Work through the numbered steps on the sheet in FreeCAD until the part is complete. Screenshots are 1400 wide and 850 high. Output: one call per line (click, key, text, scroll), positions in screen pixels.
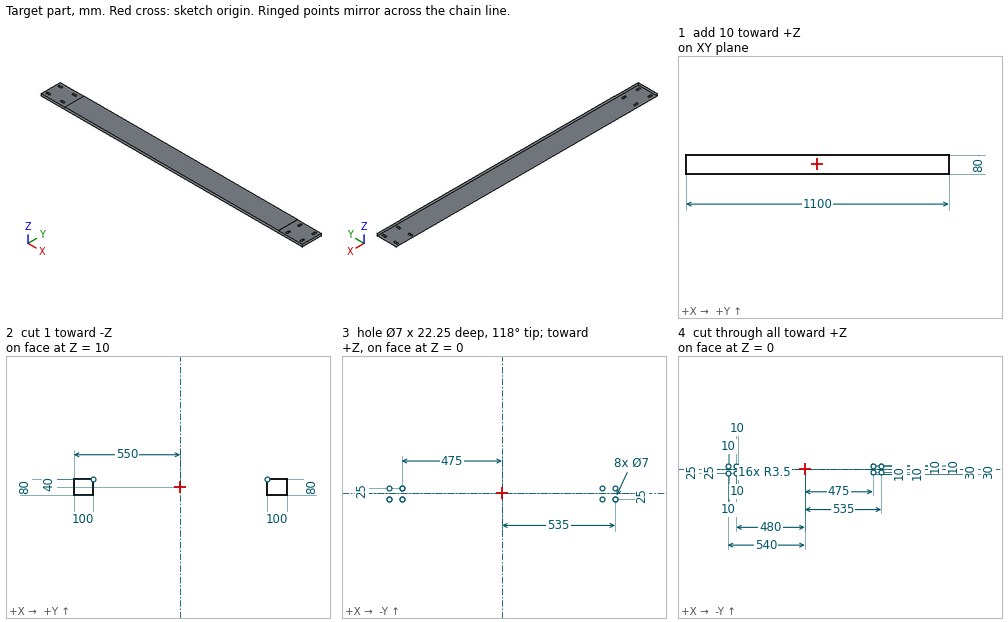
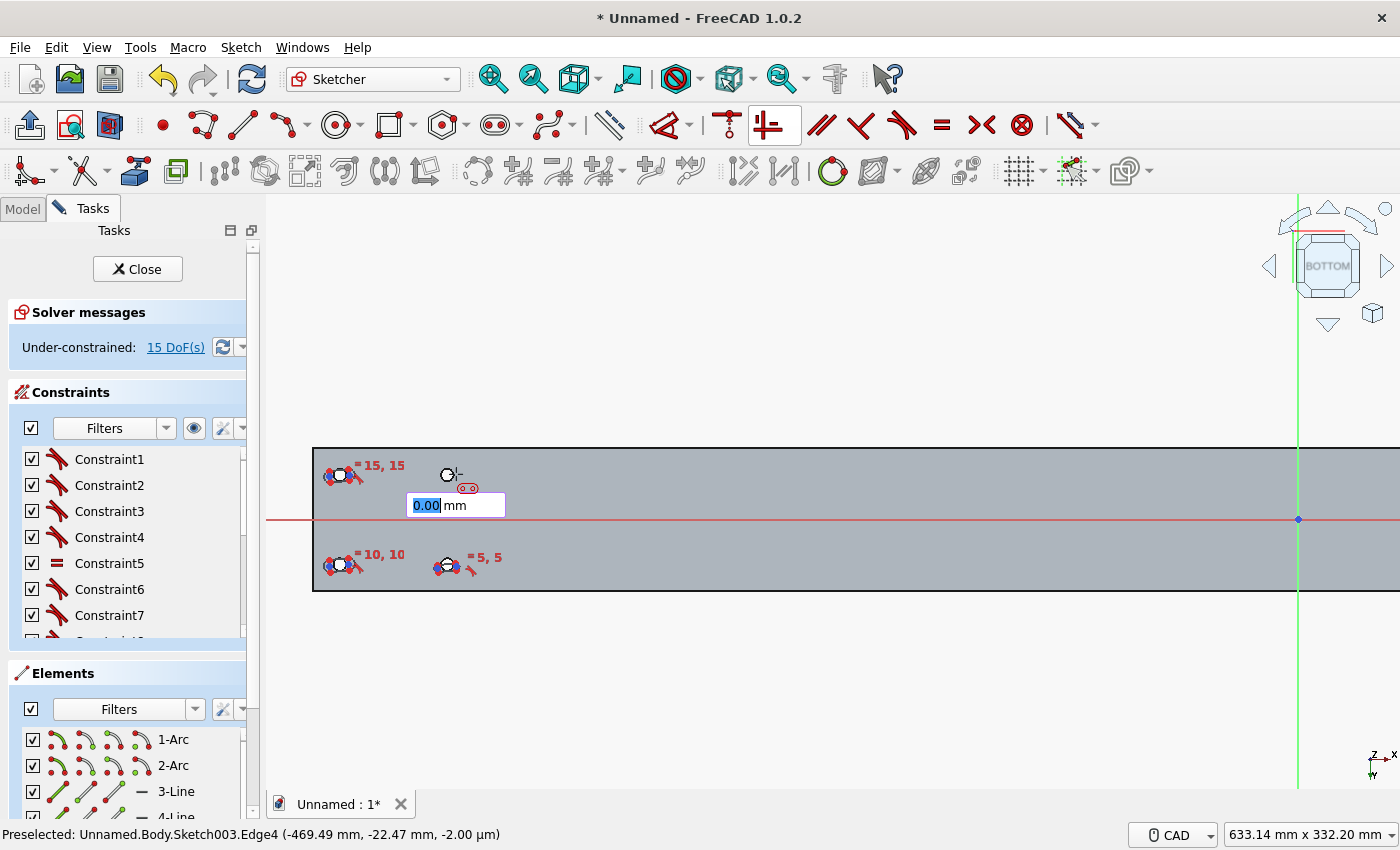
scroll(447, 481, up, 5)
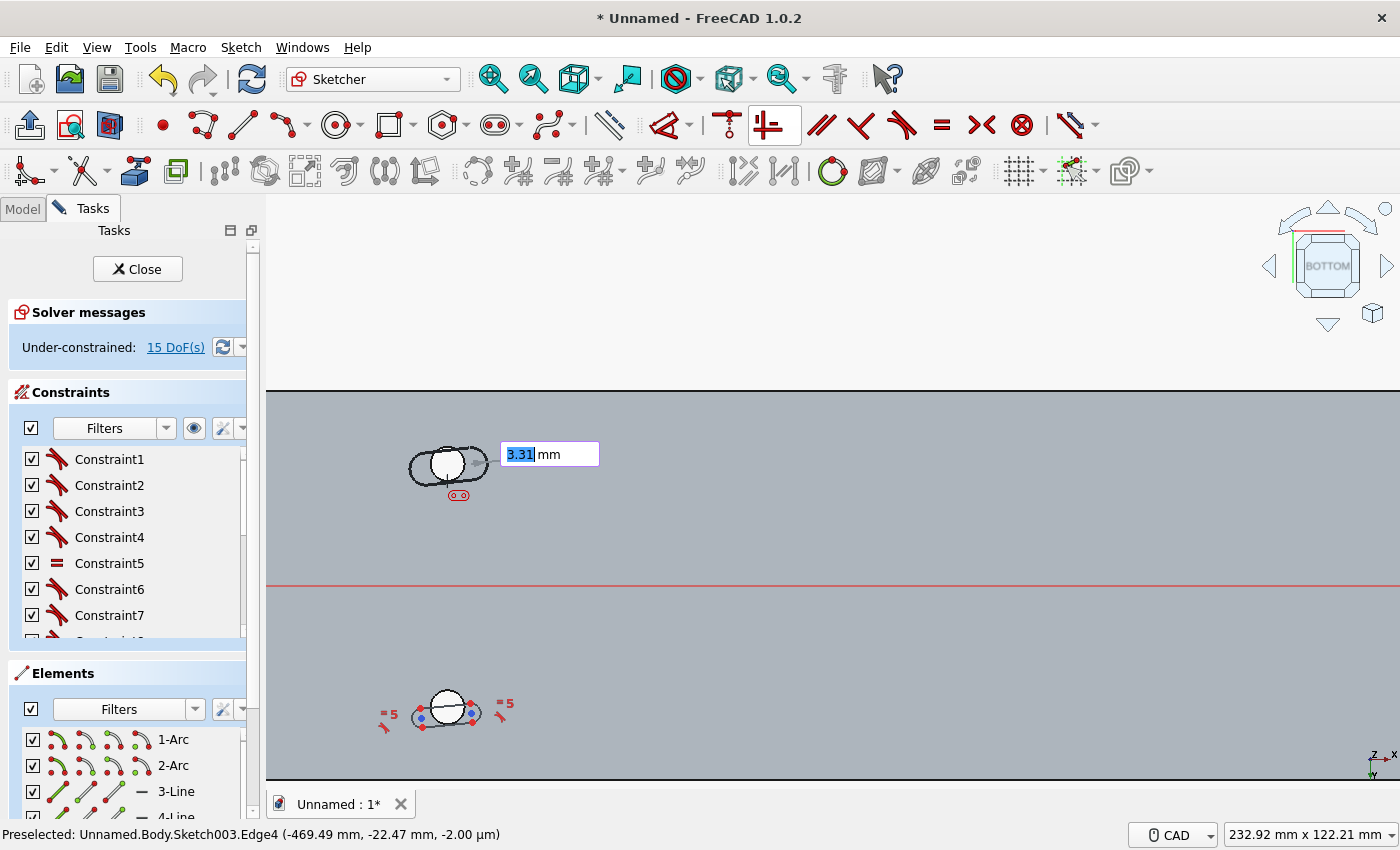
click(448, 481)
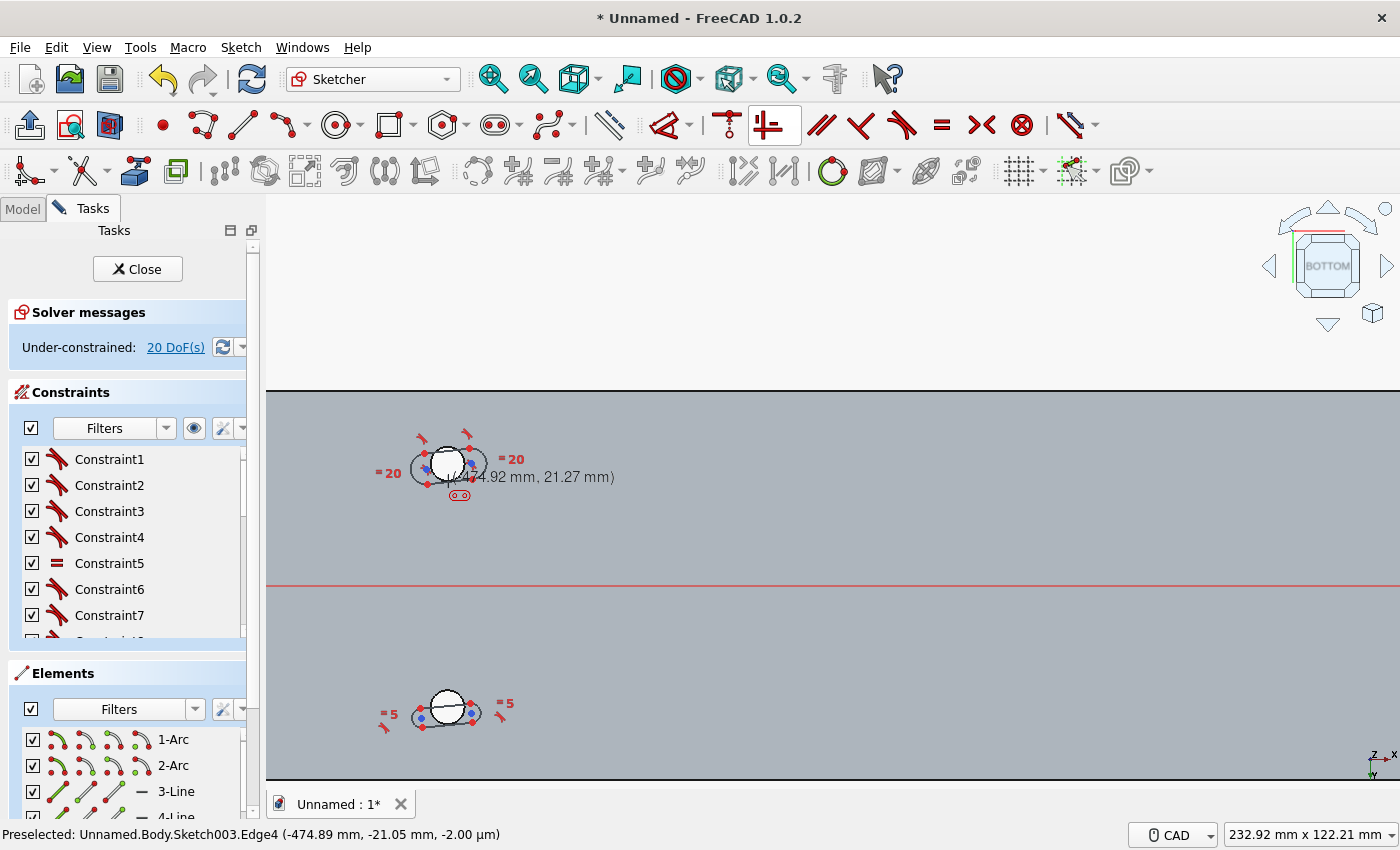
scroll(454, 477, down, 10)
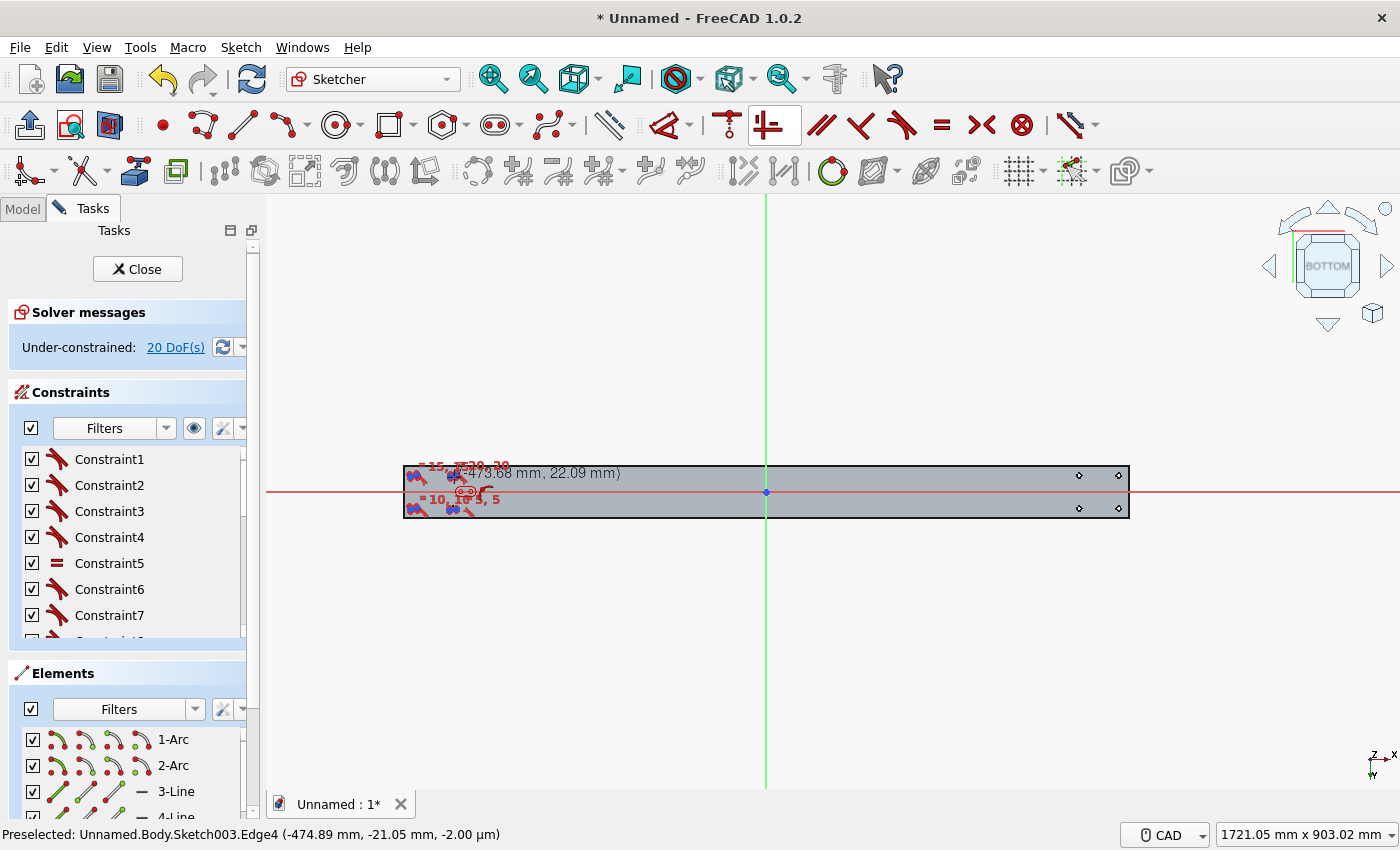
scroll(1119, 512, up, 12)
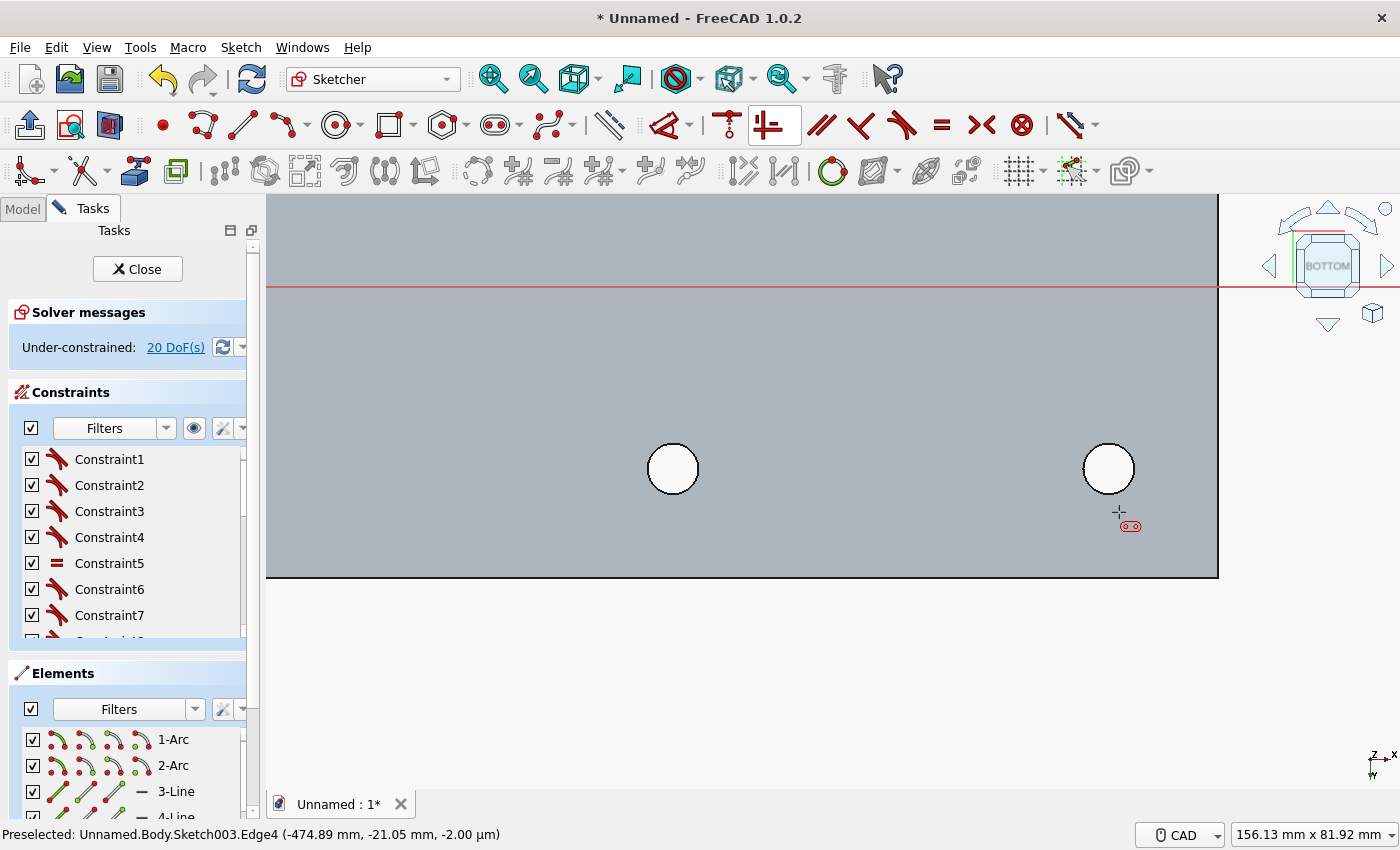
scroll(1120, 512, down, 12)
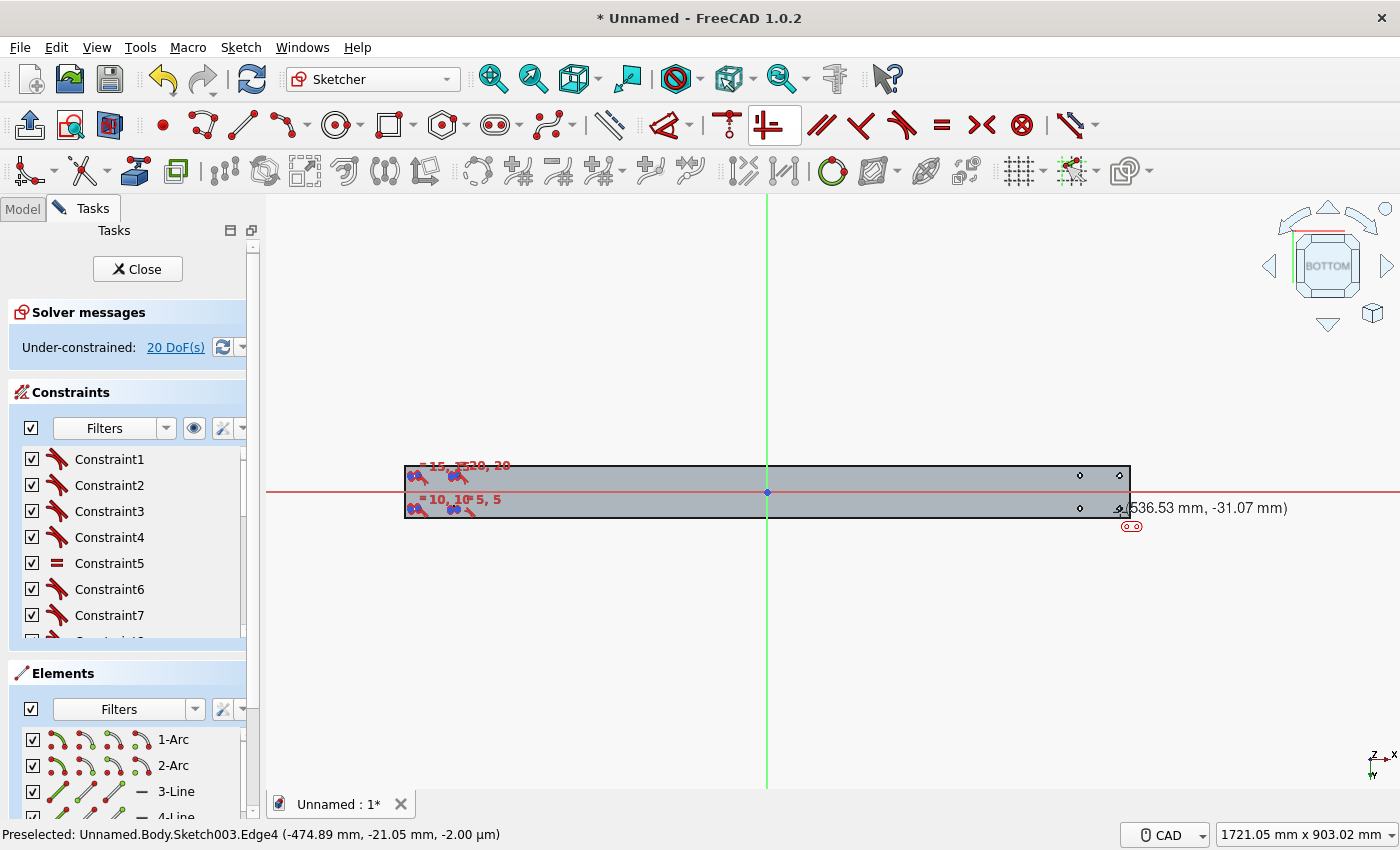
click(1120, 512)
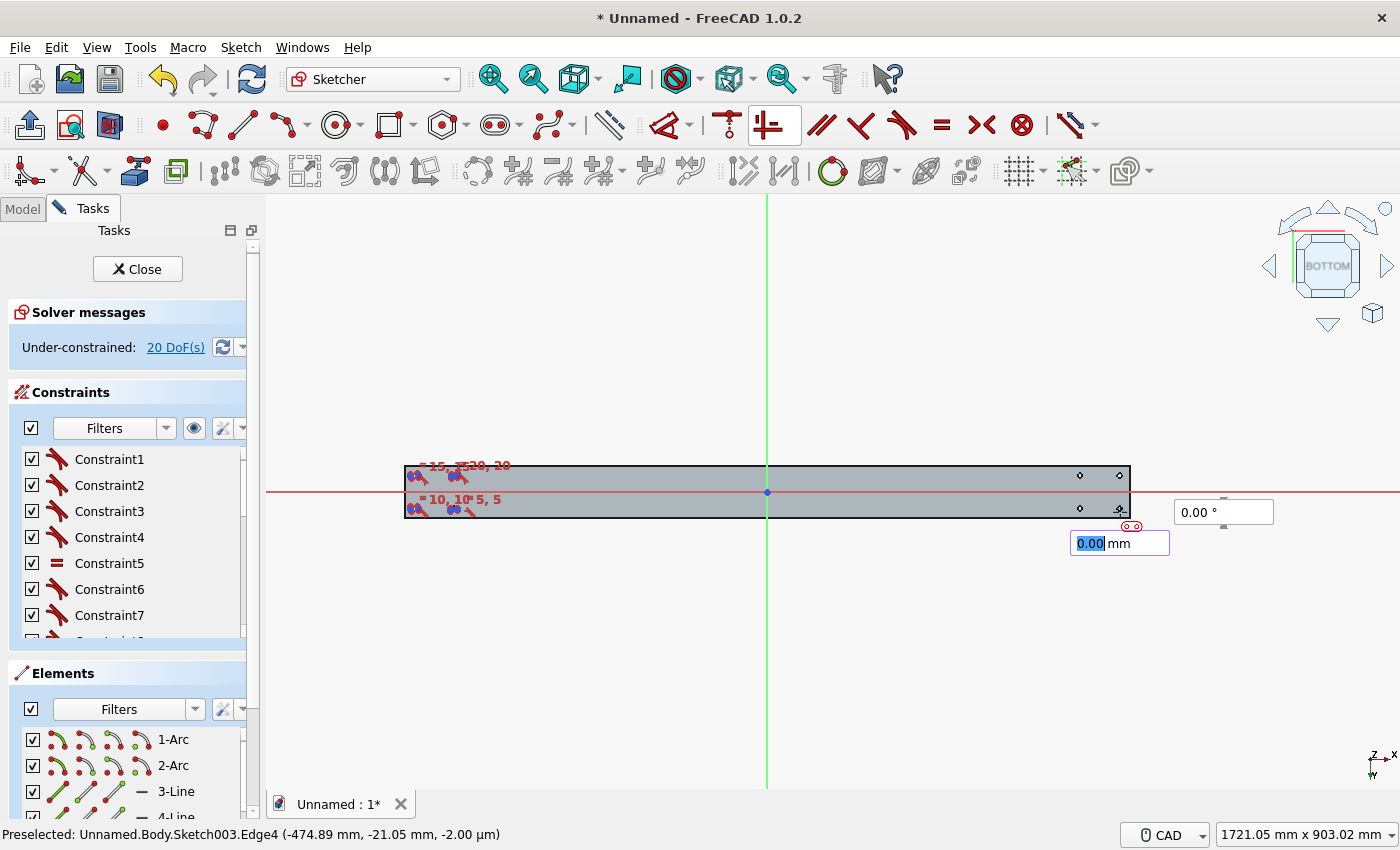
scroll(1120, 505, up, 5)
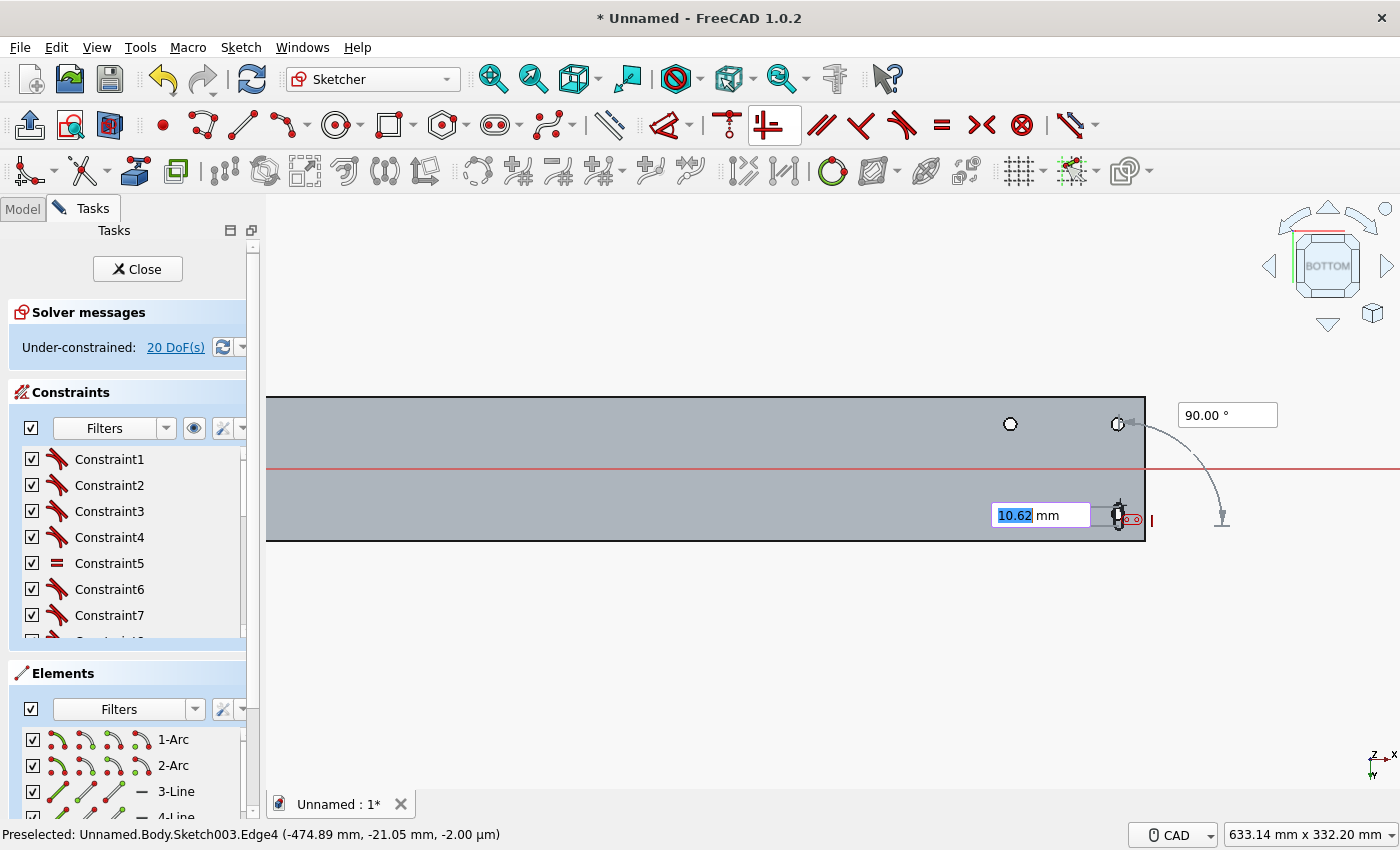
click(1119, 505)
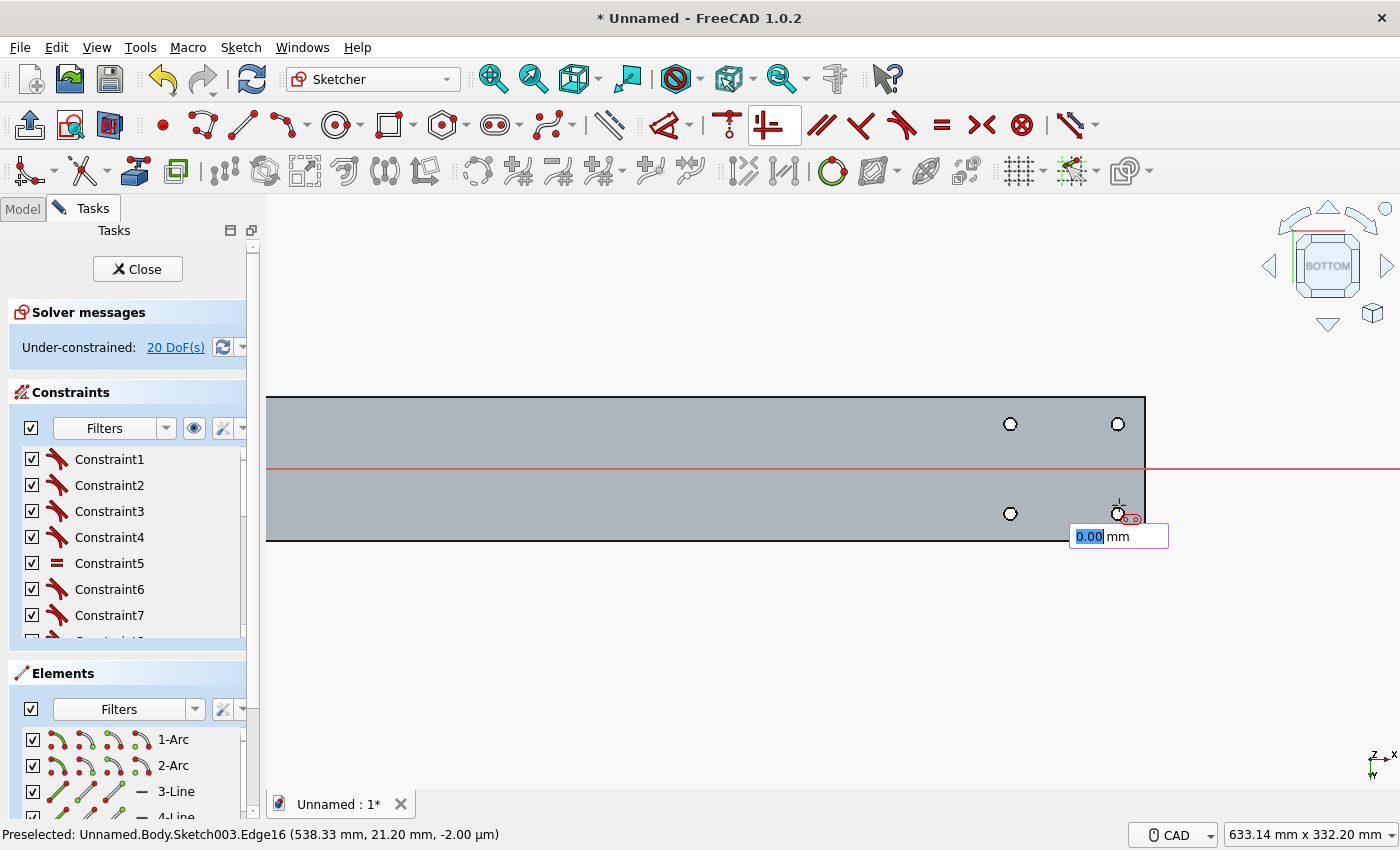
scroll(1112, 514, up, 5)